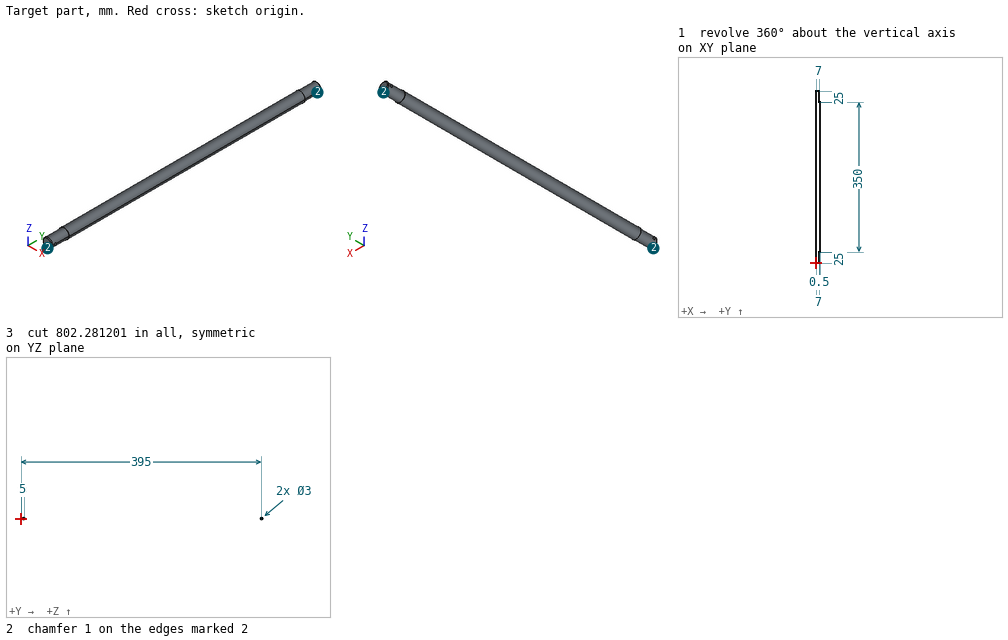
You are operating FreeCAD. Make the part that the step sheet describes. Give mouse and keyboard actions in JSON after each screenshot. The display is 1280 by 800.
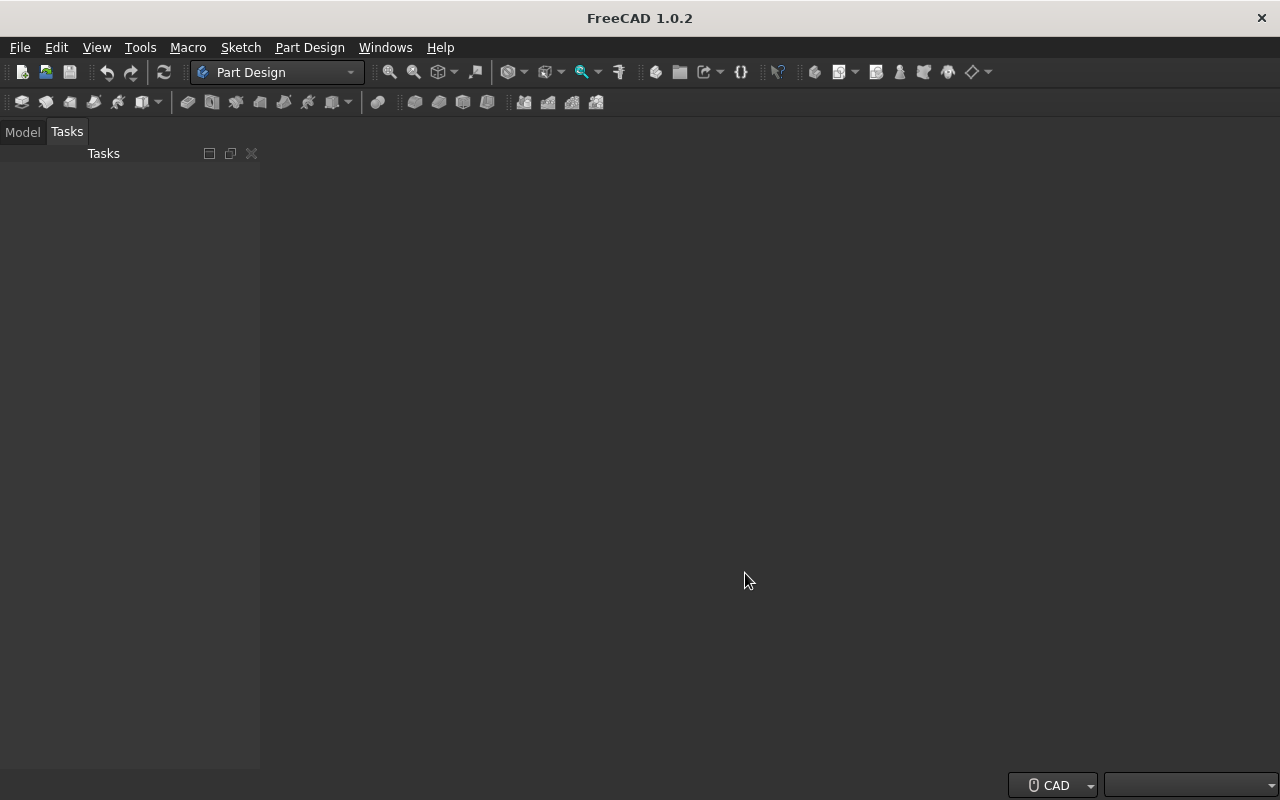
{"action": "left_click", "coordinate": [22, 72]}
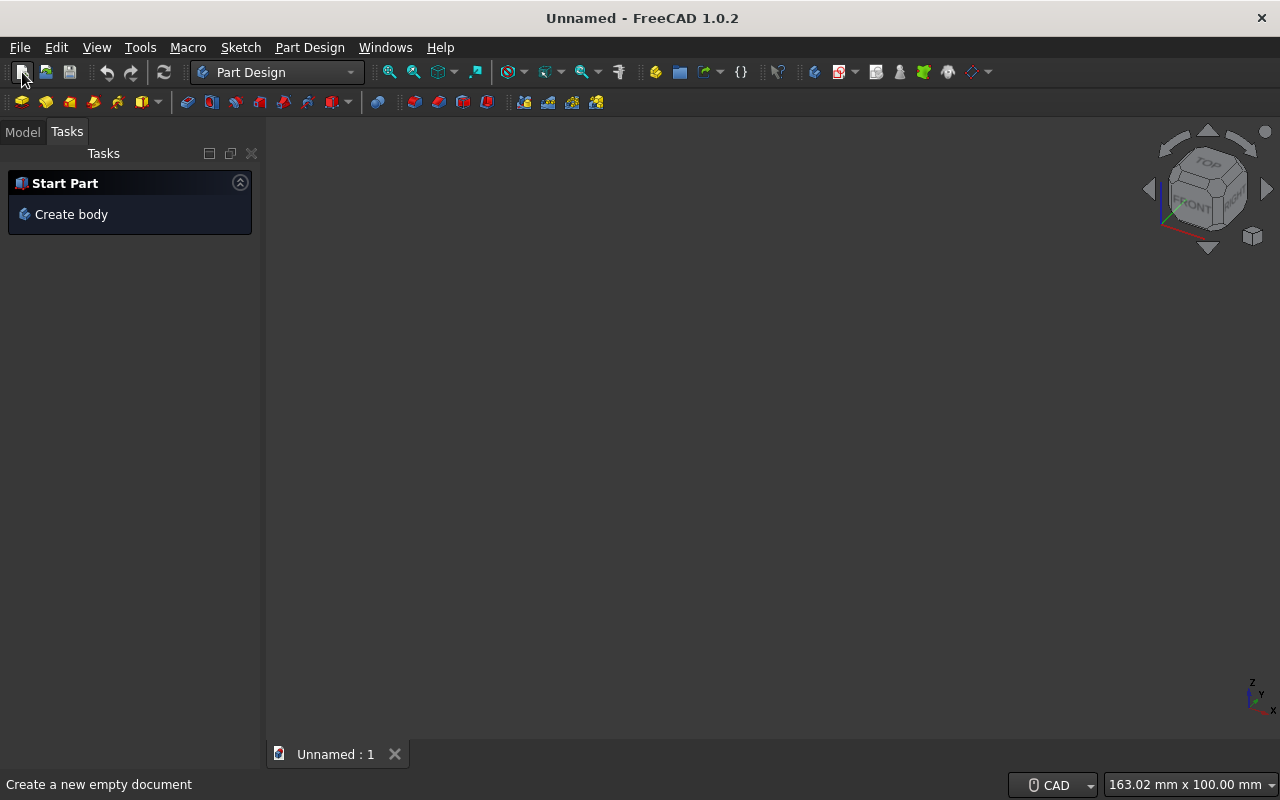
{"action": "left_click", "coordinate": [840, 72]}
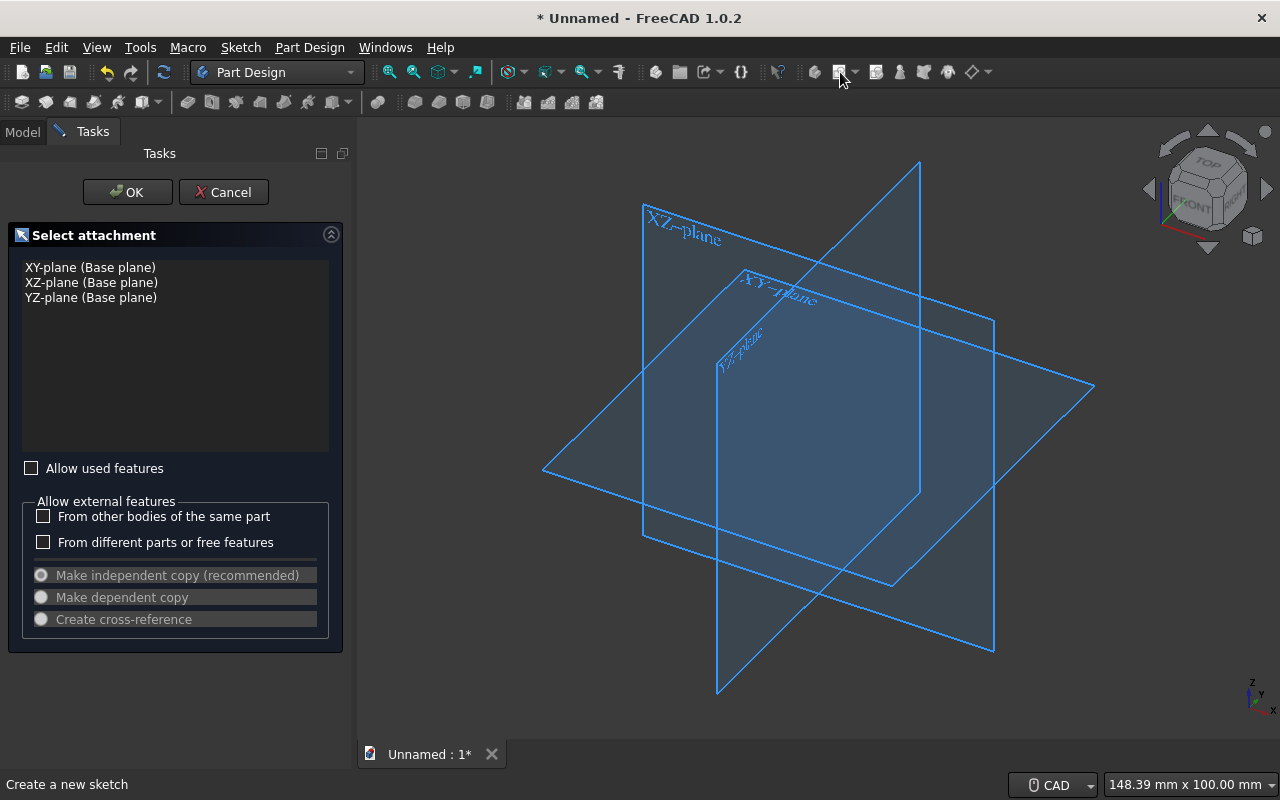
{"action": "left_click", "coordinate": [82, 268]}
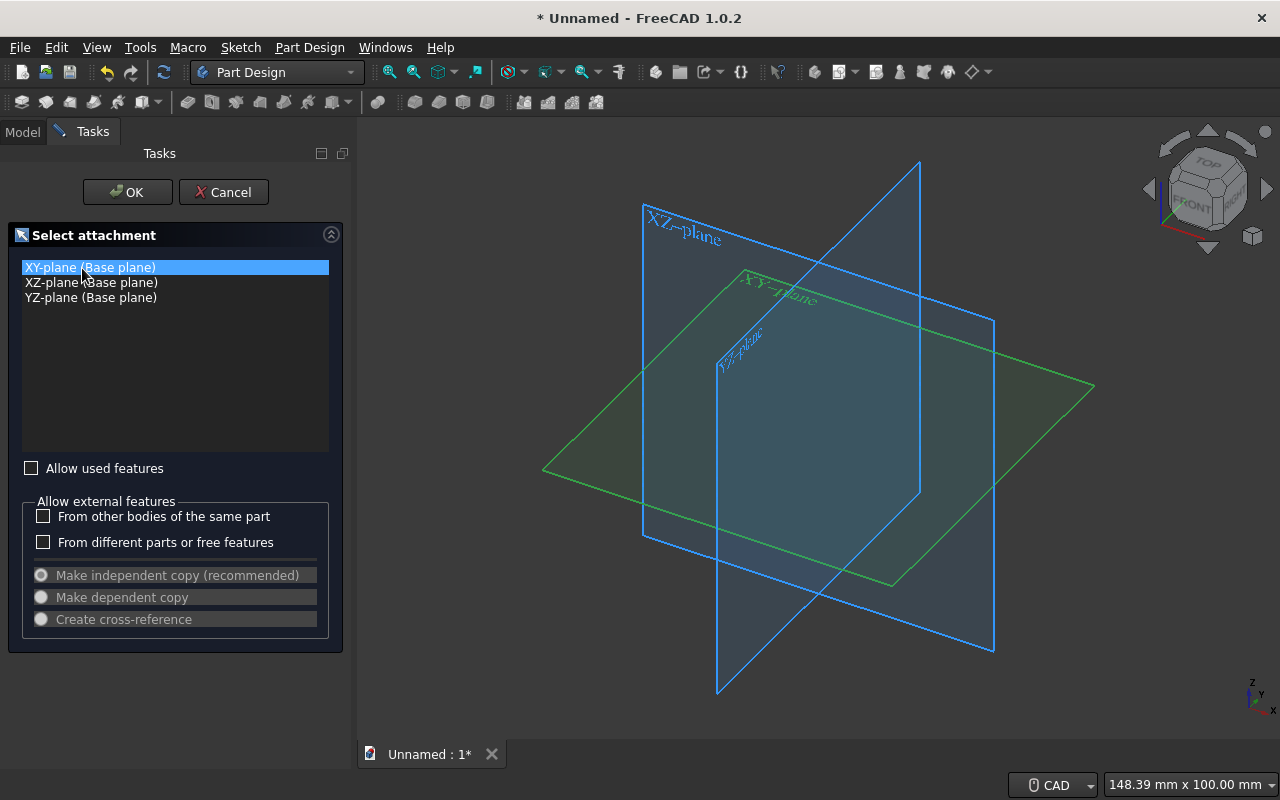
{"action": "left_click", "coordinate": [128, 192]}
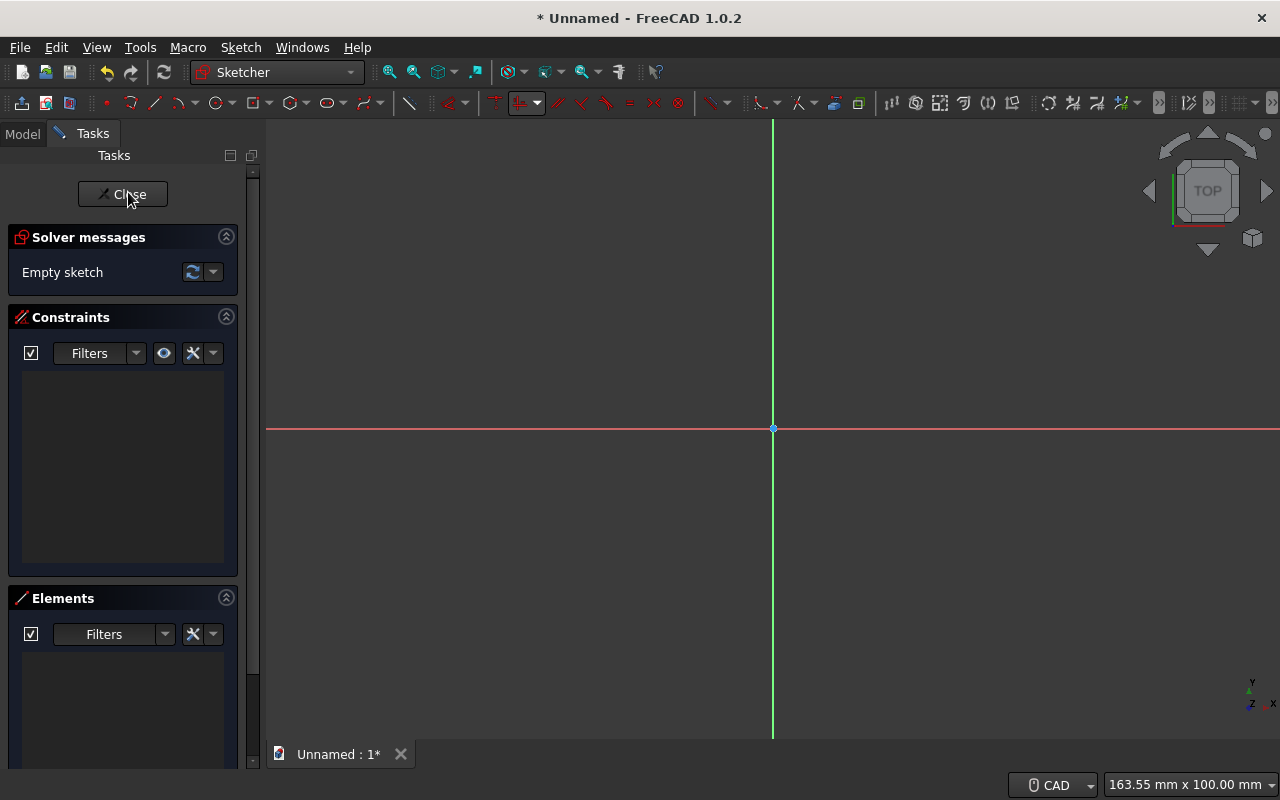
{"action": "scroll", "coordinate": [686, 675], "scroll_direction": "down", "scroll_amount": 9}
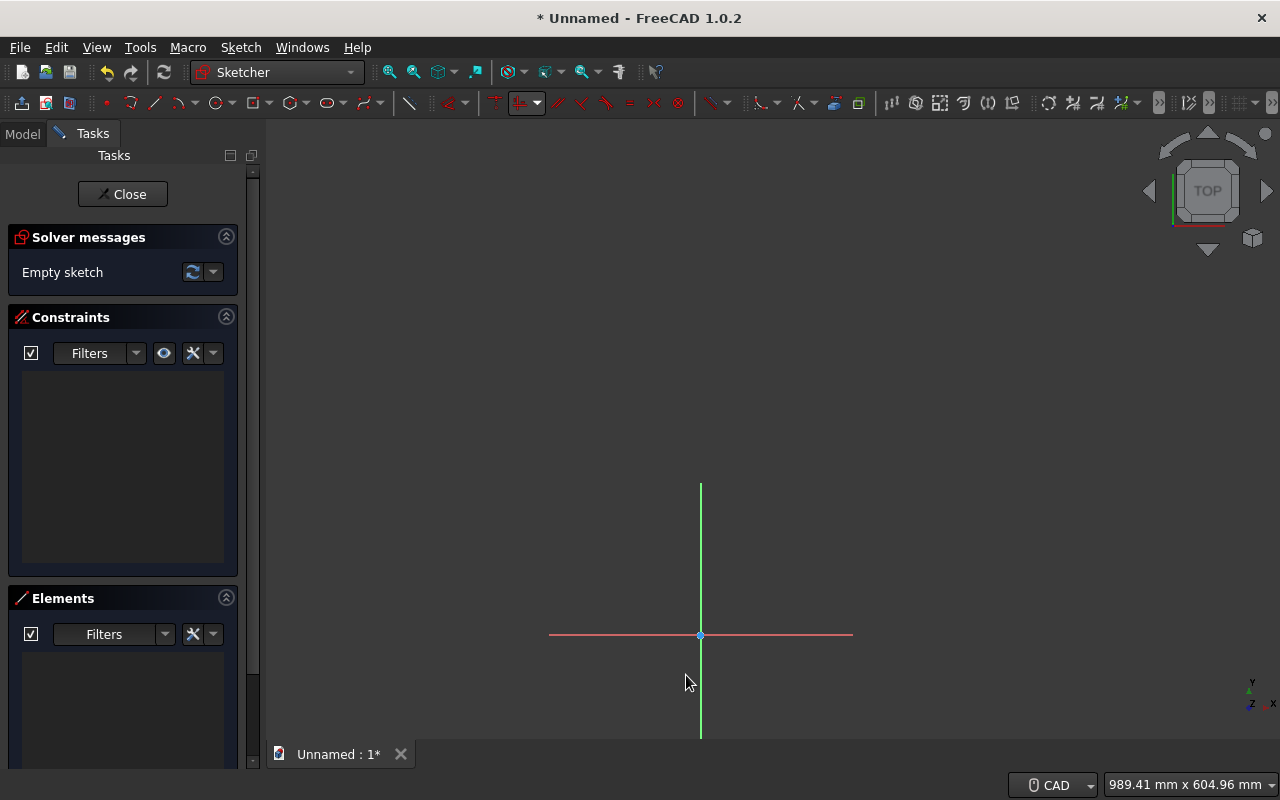
{"action": "key", "text": "g m"}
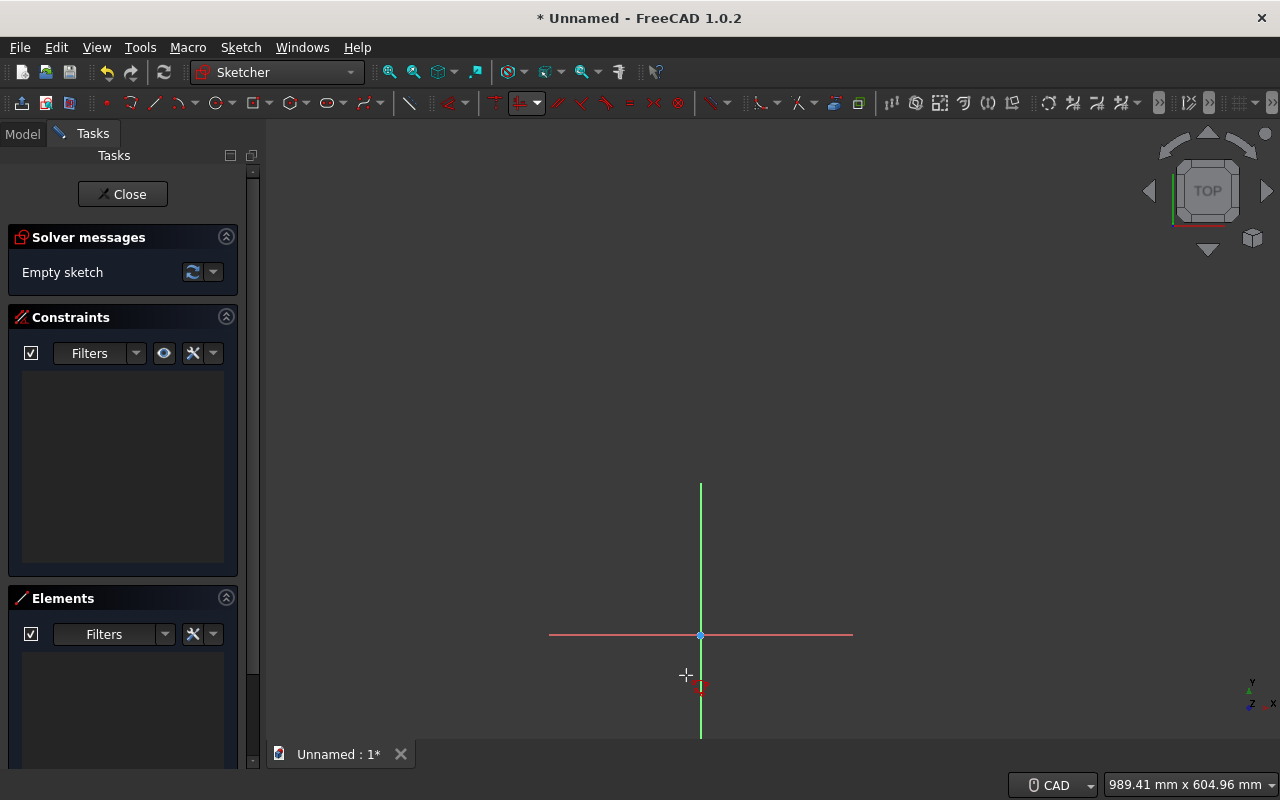
{"action": "left_click", "coordinate": [701, 635]}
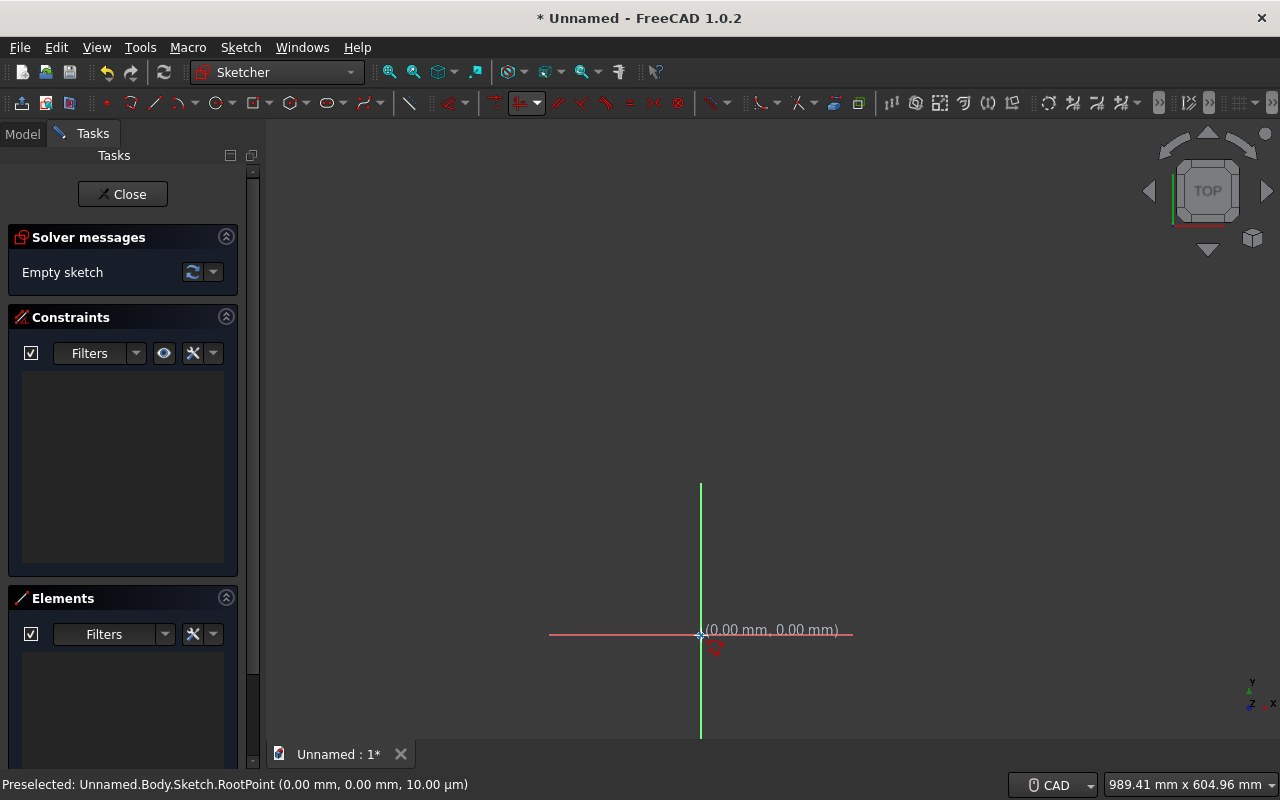
{"action": "scroll", "coordinate": [708, 635], "scroll_direction": "up", "scroll_amount": 4}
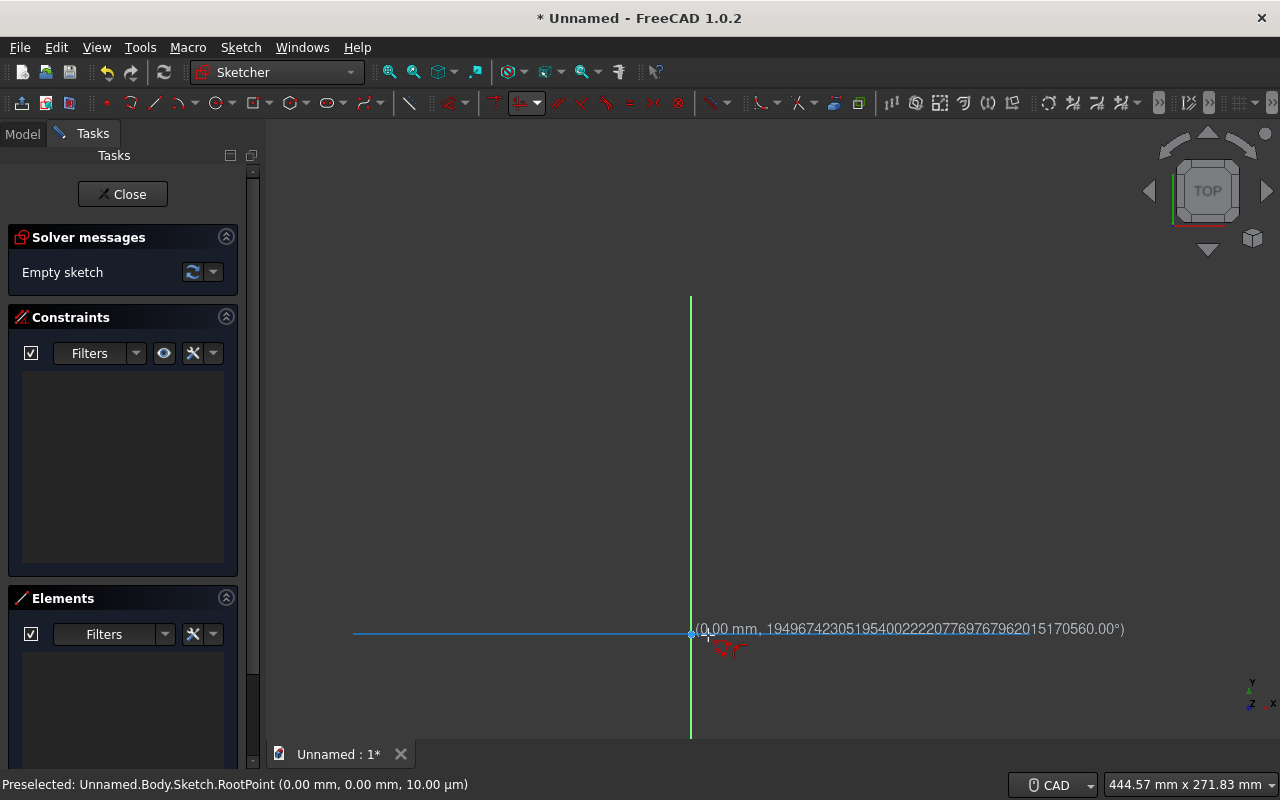
{"action": "left_click", "coordinate": [707, 625]}
{"action": "left_click", "coordinate": [707, 577]}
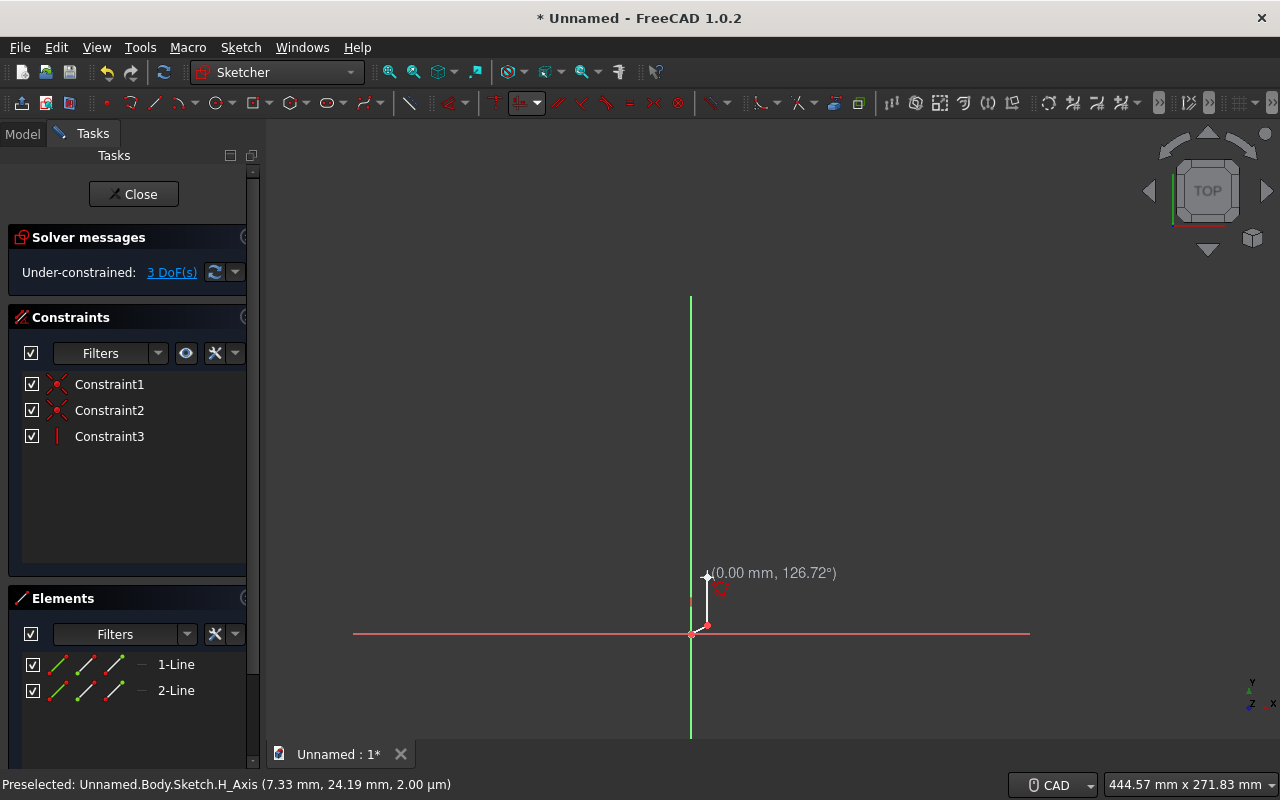
{"action": "scroll", "coordinate": [708, 577], "scroll_direction": "up", "scroll_amount": 14}